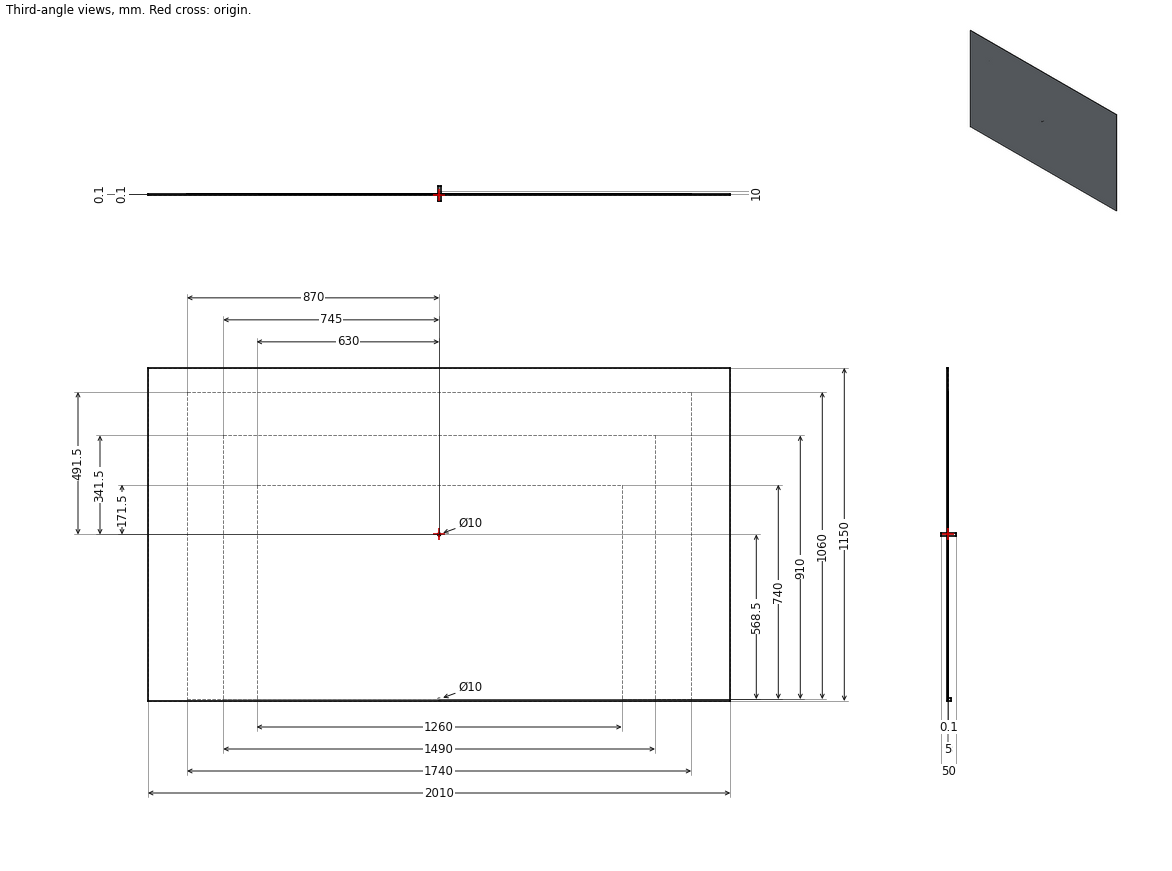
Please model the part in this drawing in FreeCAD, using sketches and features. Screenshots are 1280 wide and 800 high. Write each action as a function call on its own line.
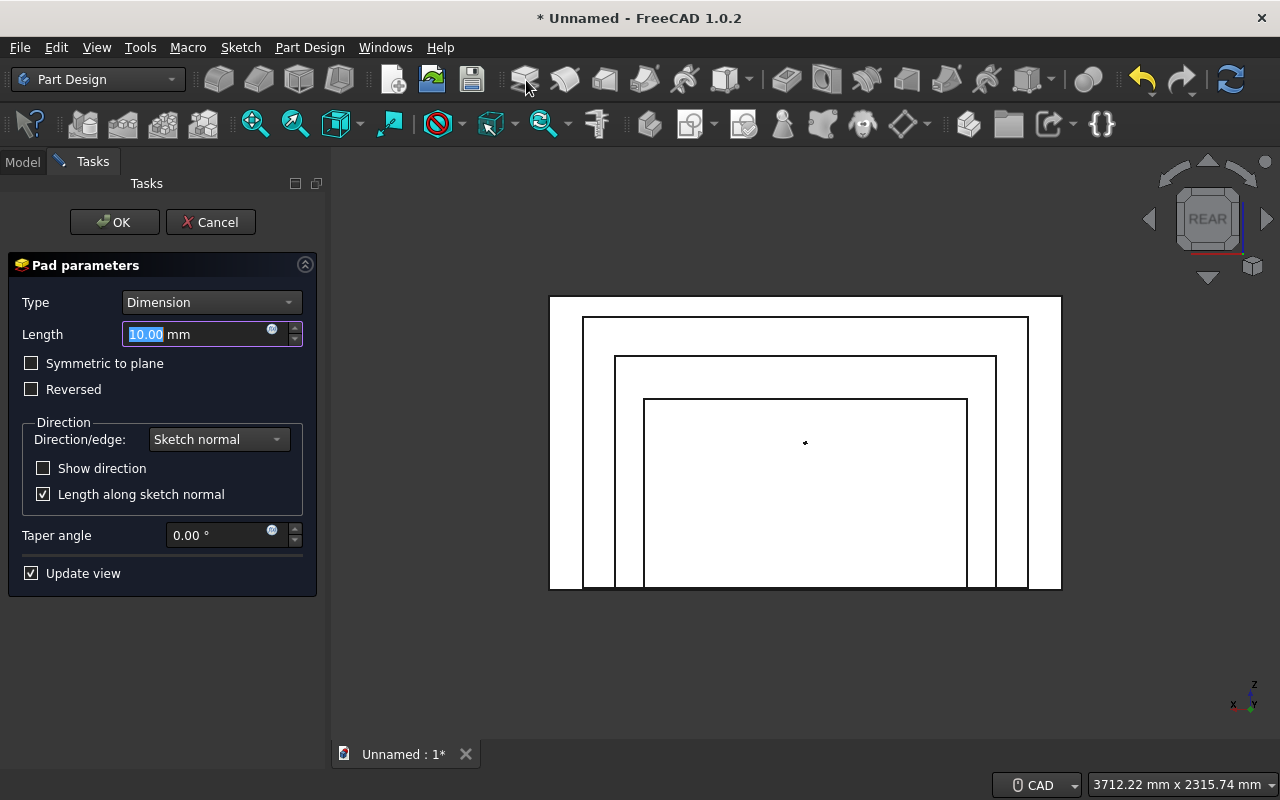
text(50)
key(Tab)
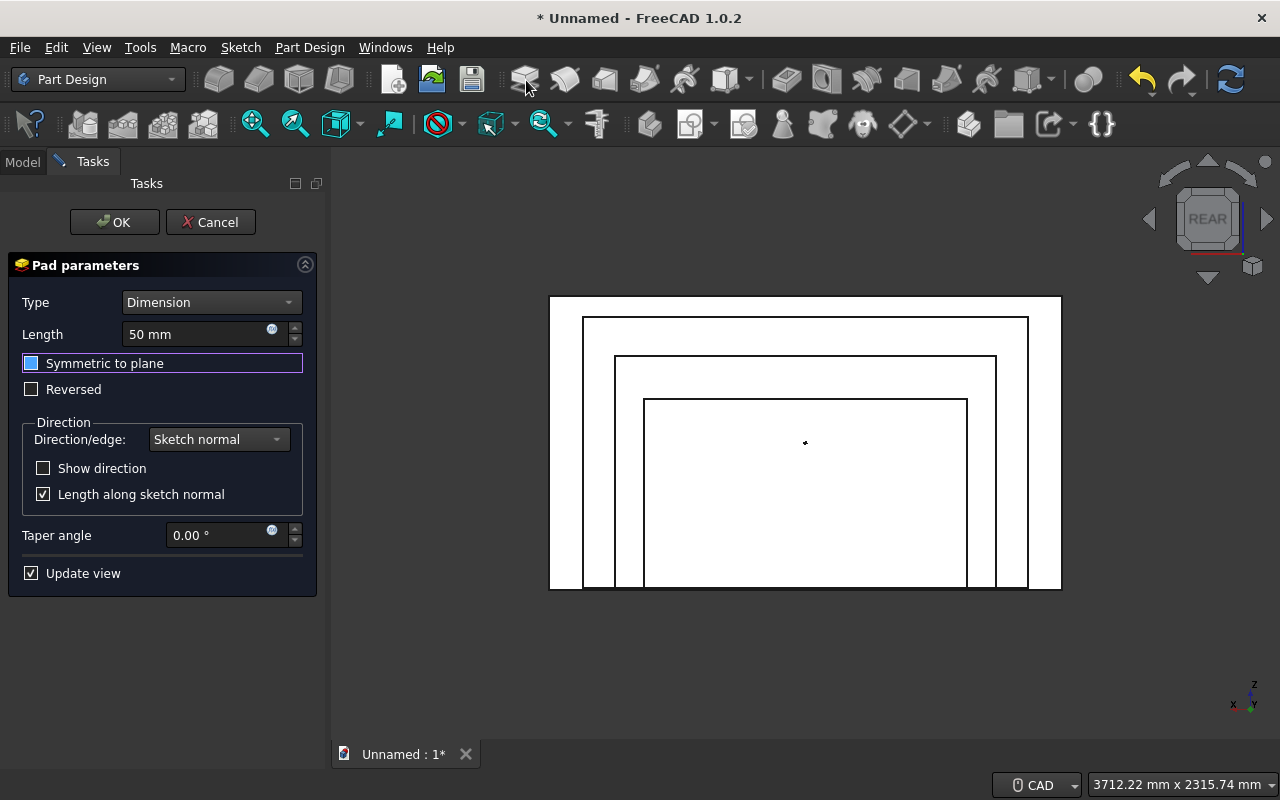
click(30, 363)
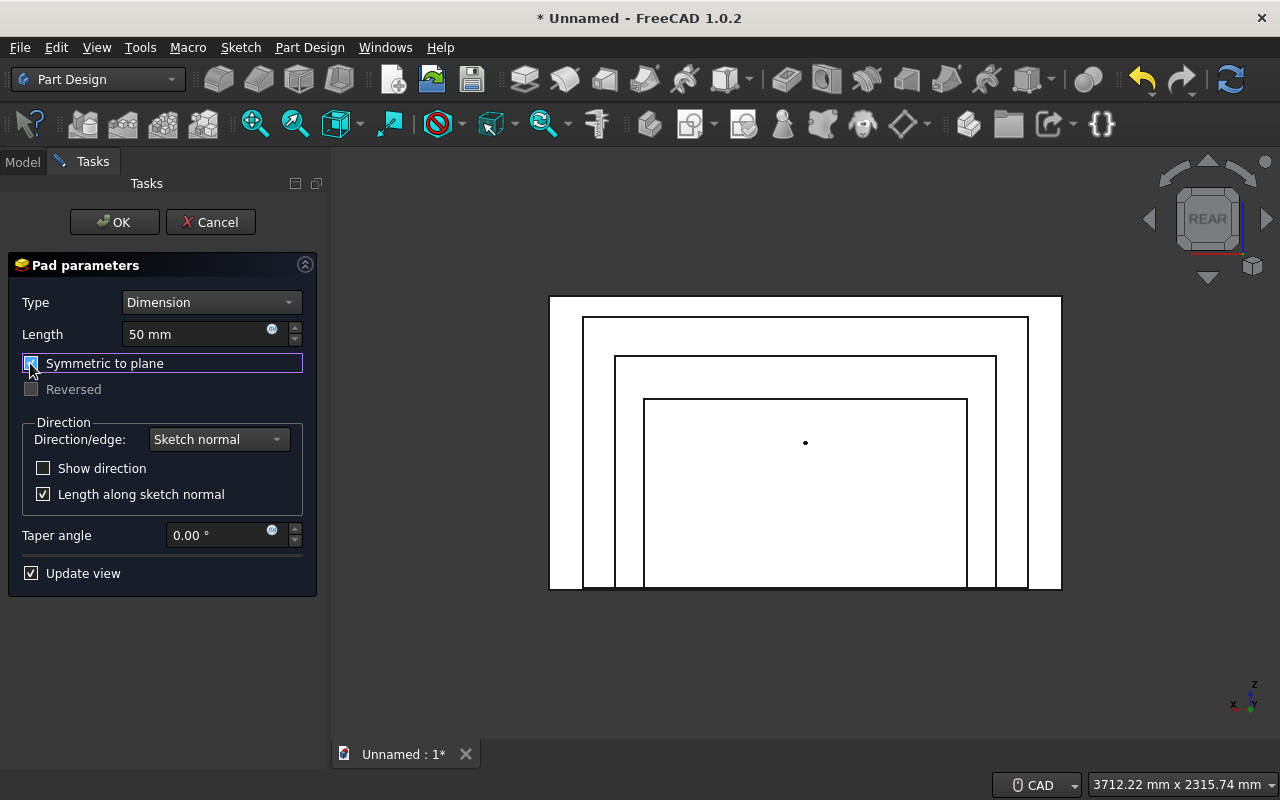
click(115, 222)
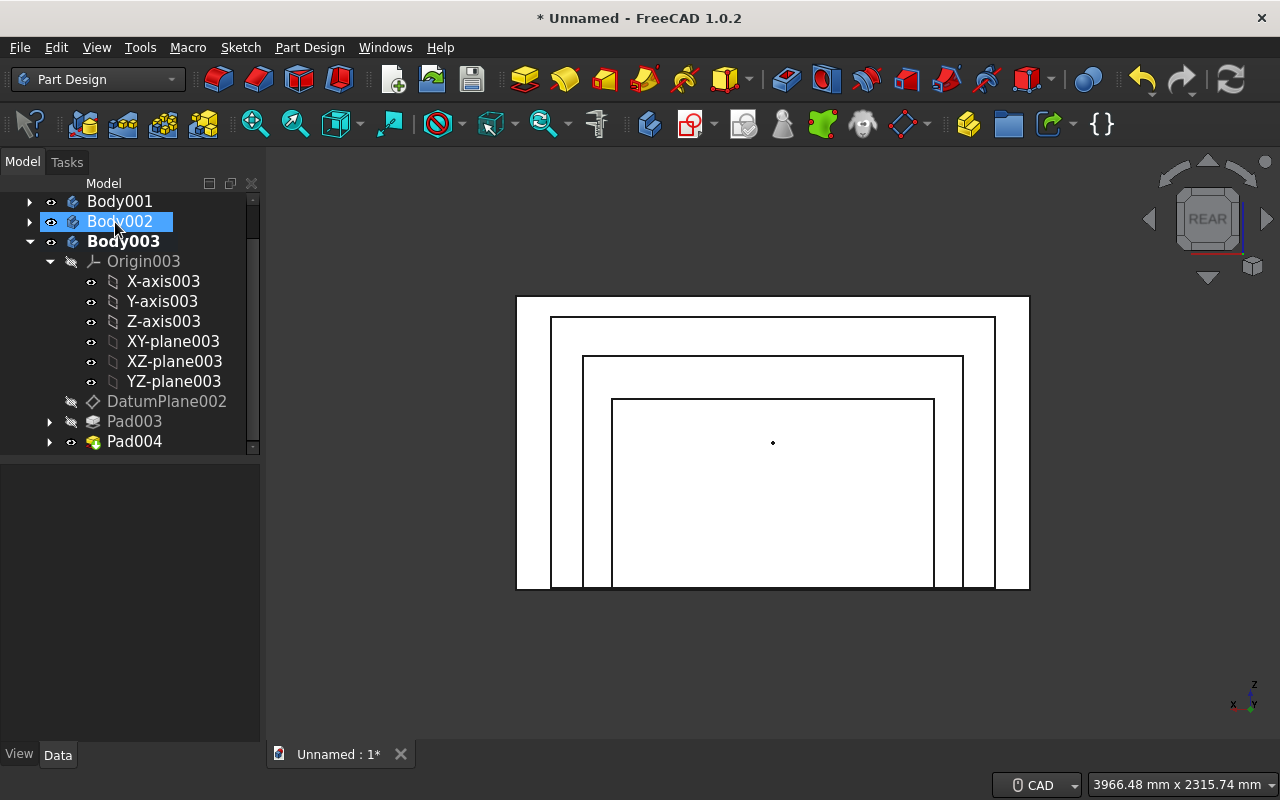
click(256, 124)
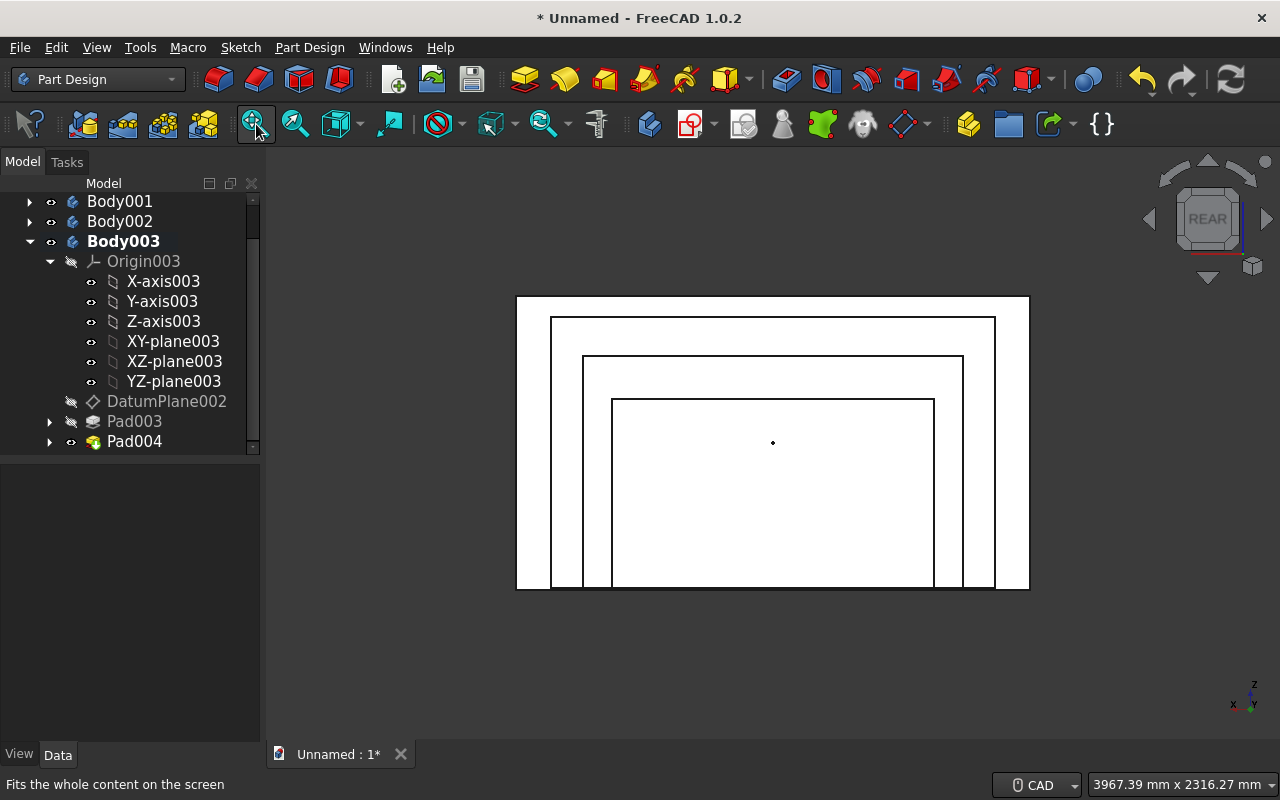
click(681, 493)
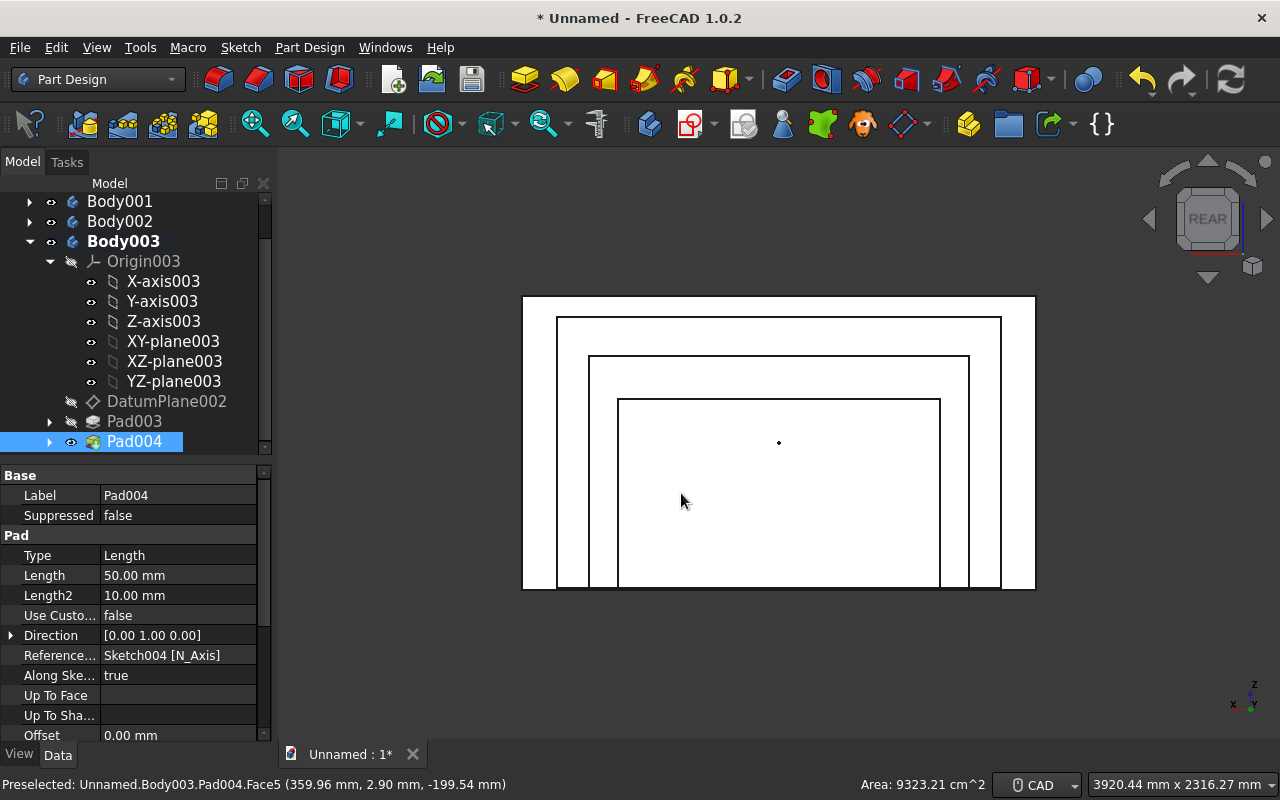
click(690, 124)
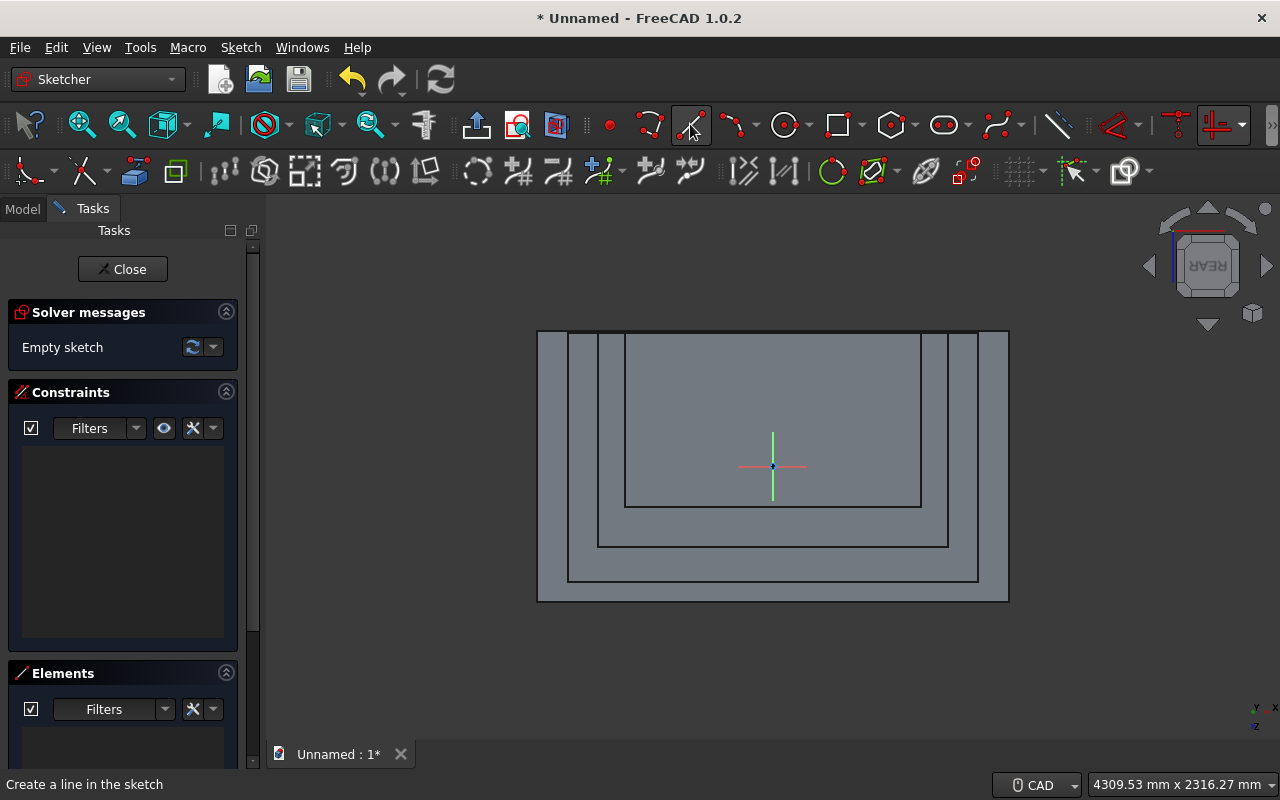
click(558, 126)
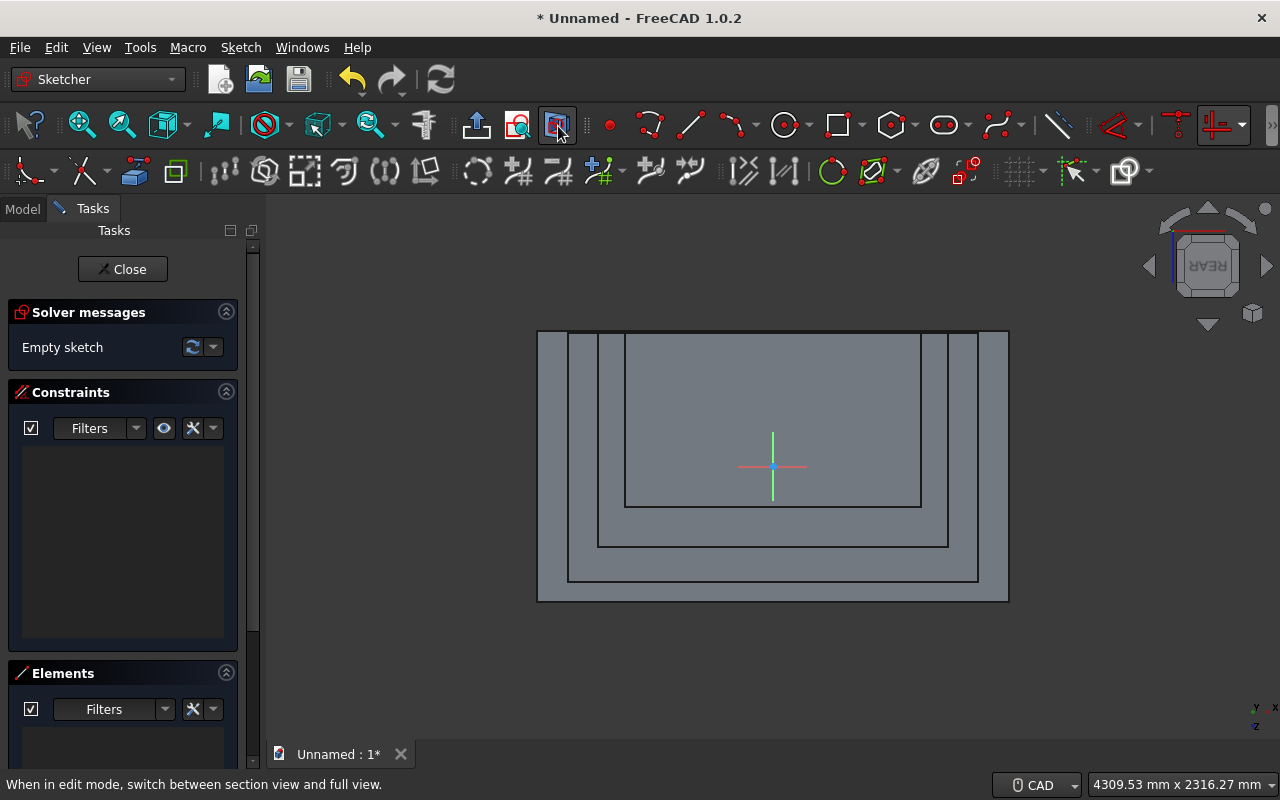
scroll(777, 326, up, 15)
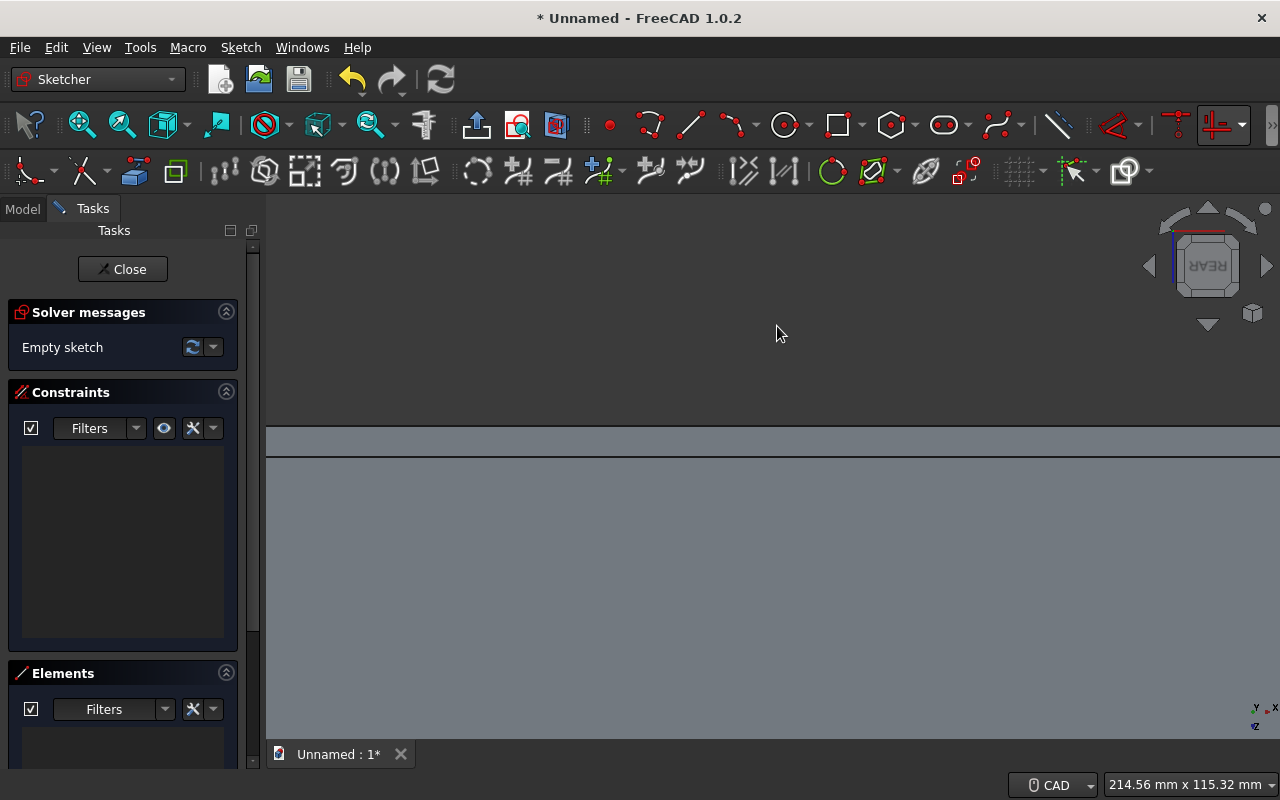
scroll(684, 455, up, 10)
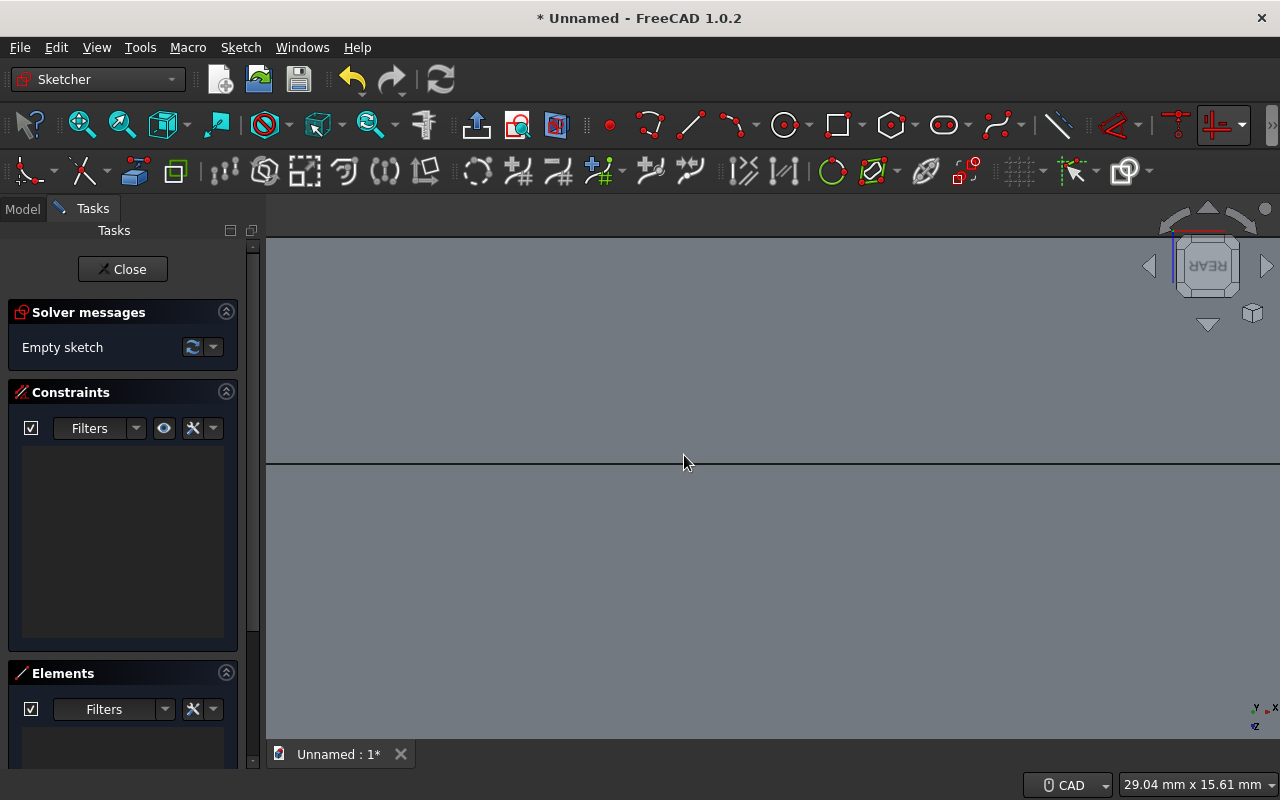
click(786, 126)